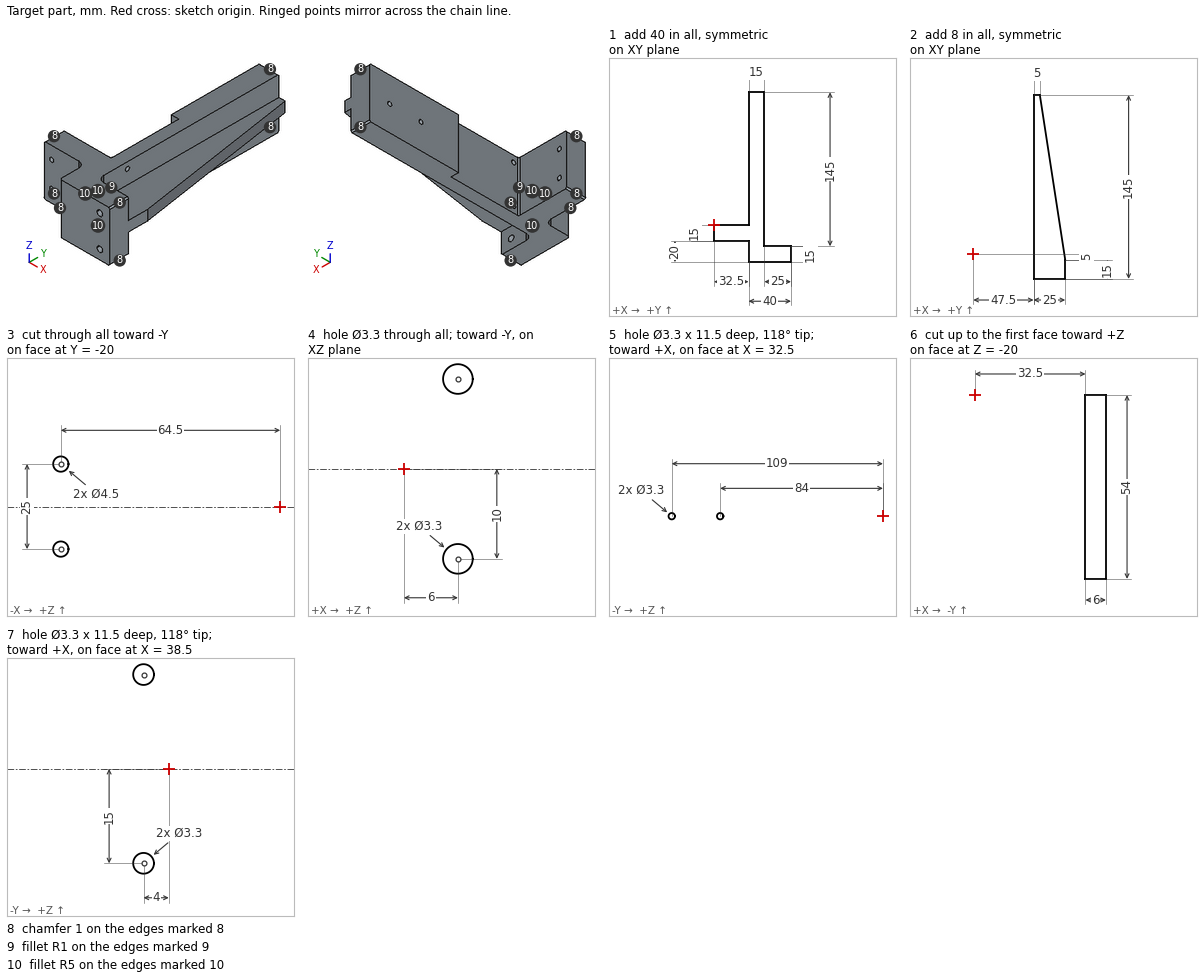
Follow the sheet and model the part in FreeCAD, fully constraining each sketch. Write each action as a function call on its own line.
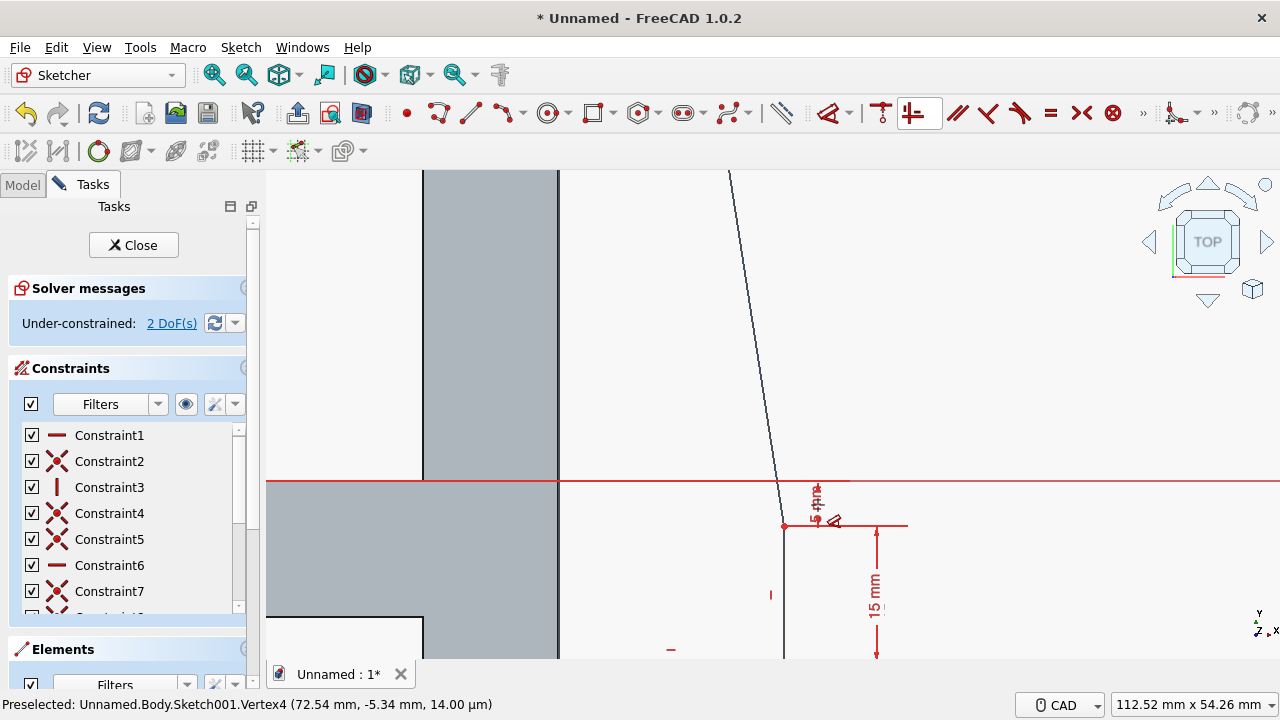
scroll(786, 547, down, 7)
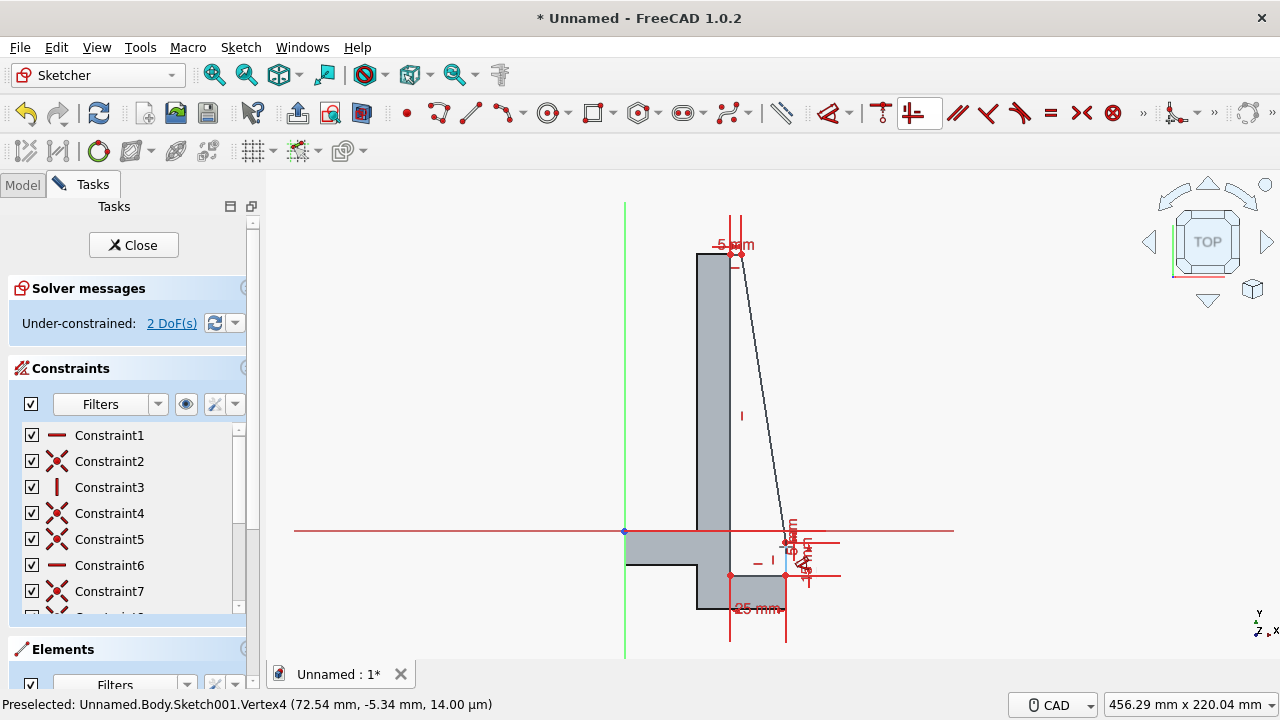
click(730, 480)
click(764, 489)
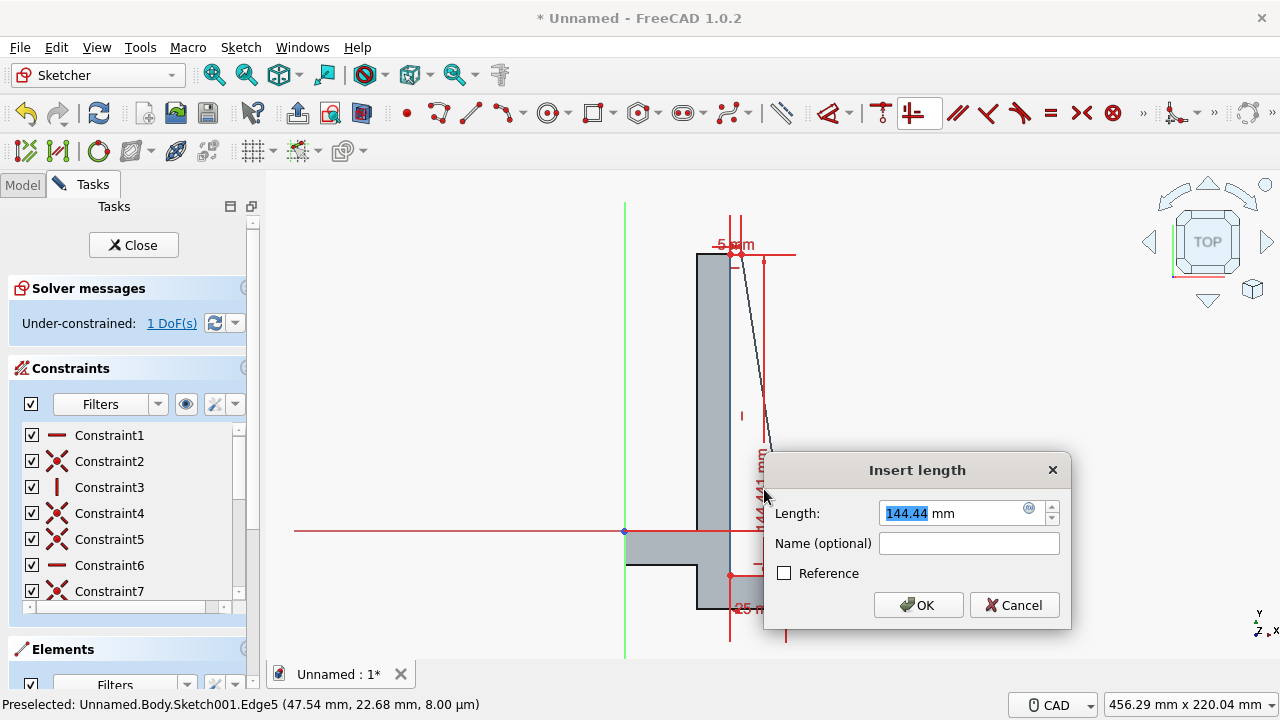
text(145)
key(Return)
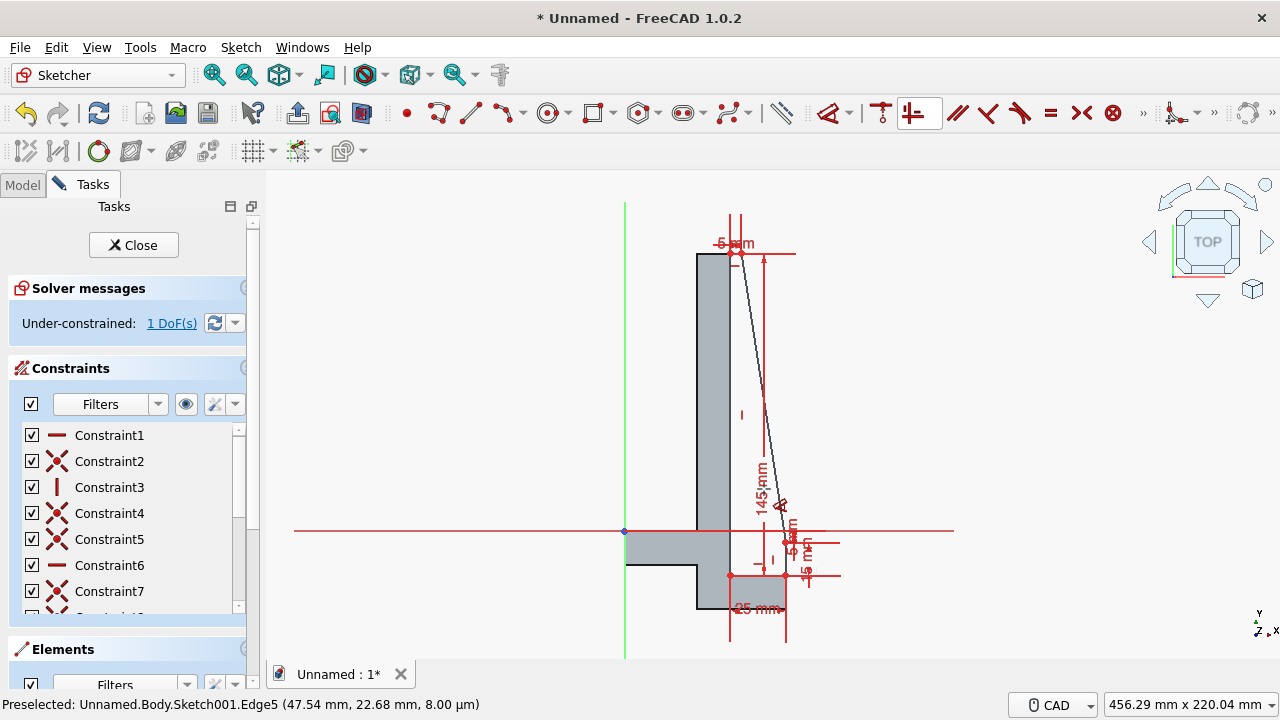
click(730, 576)
click(678, 610)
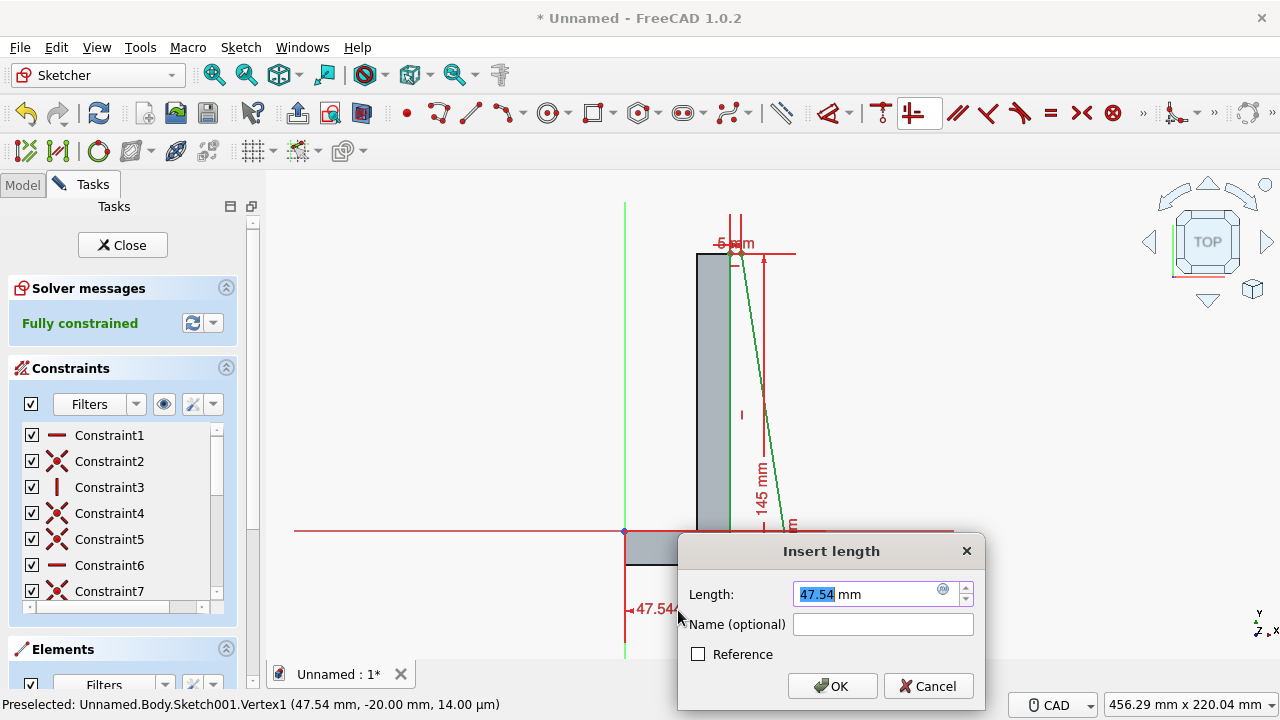
text(47.5)
key(Return)
key(Escape)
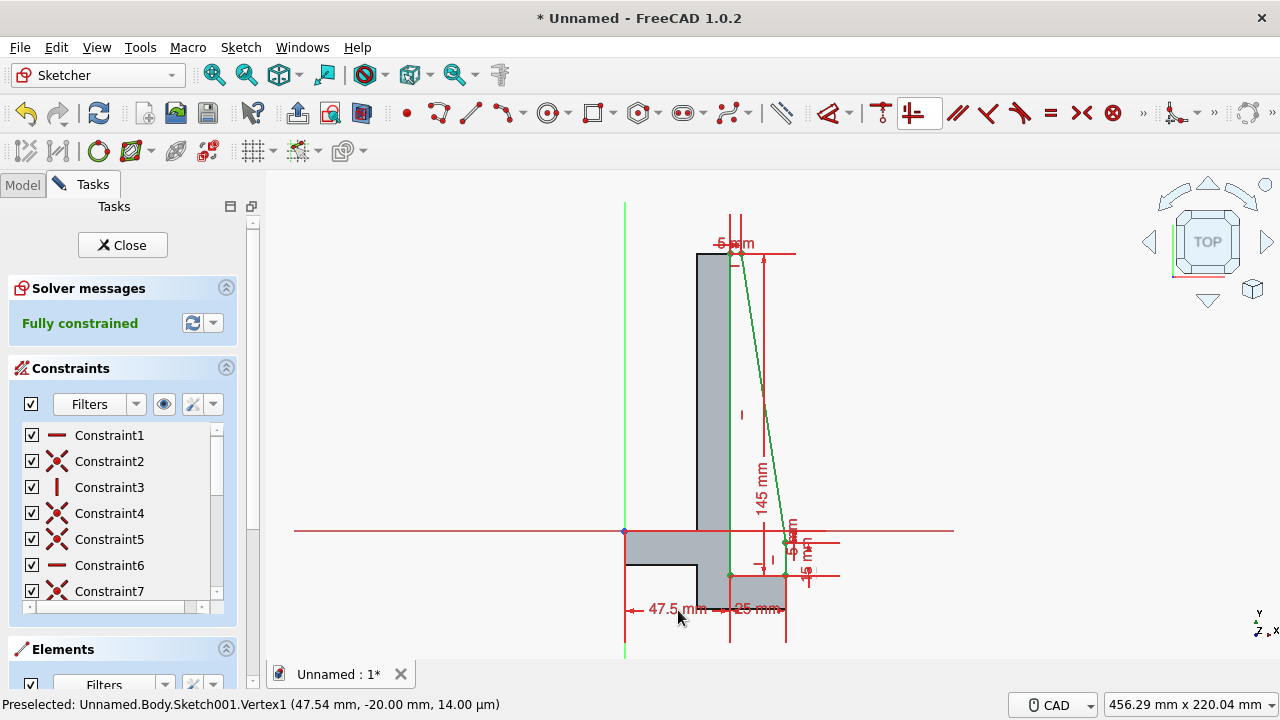
click(123, 245)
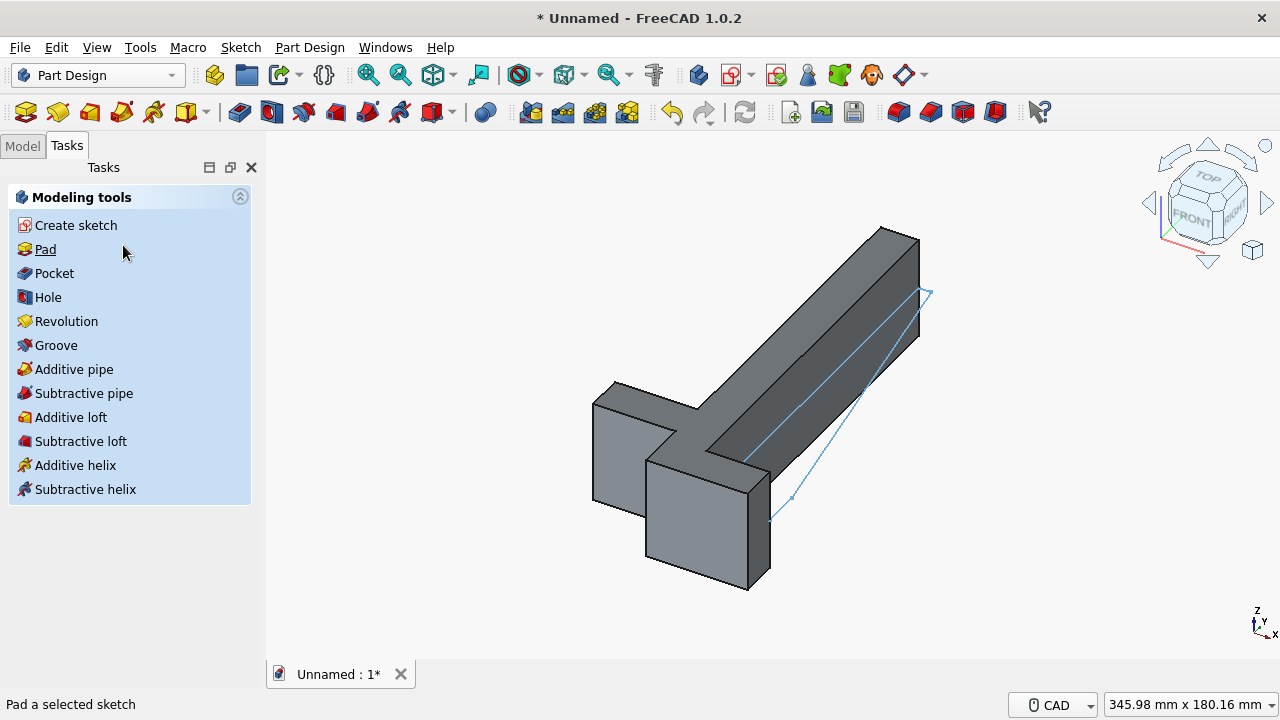
click(26, 112)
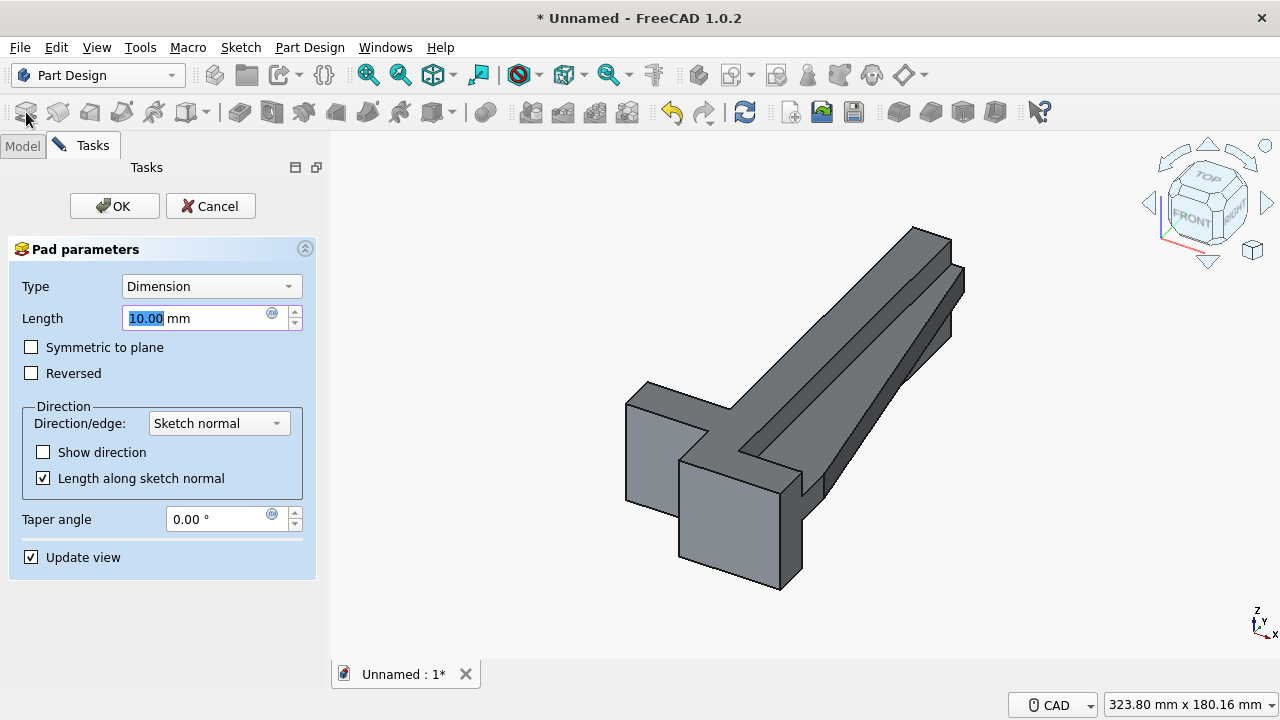
text(8)
key(Tab)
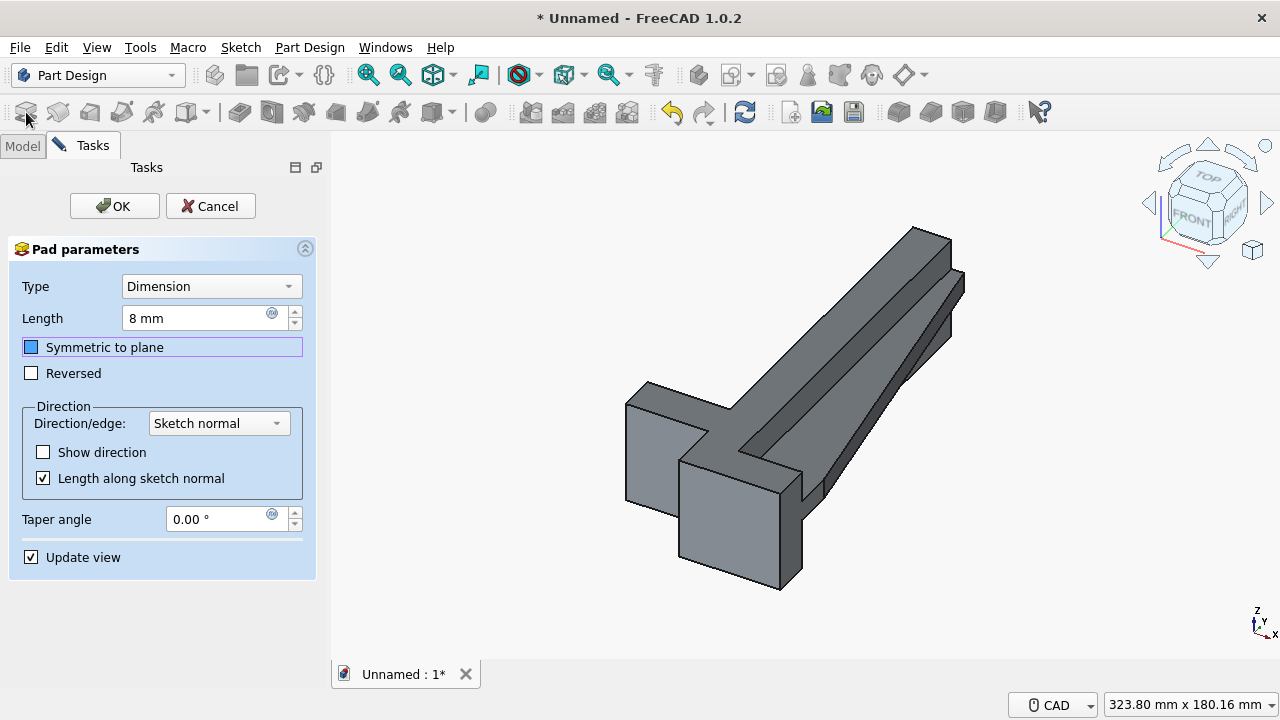
click(30, 347)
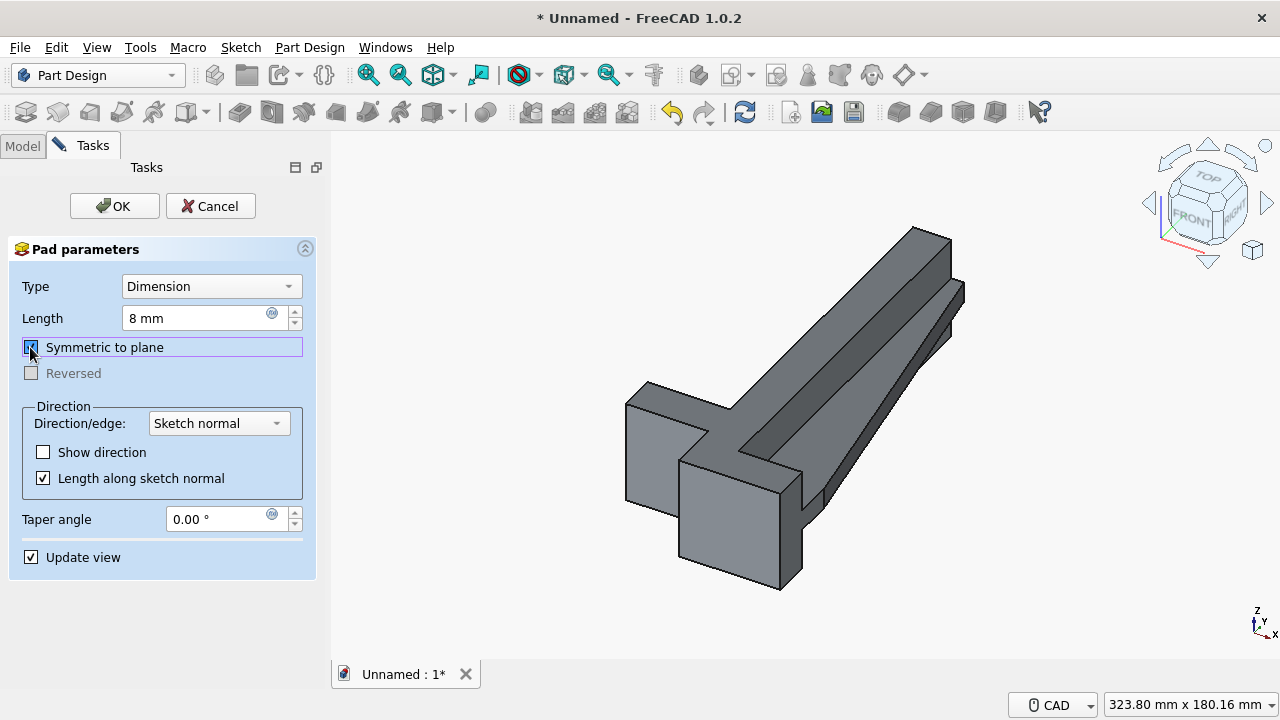
click(115, 206)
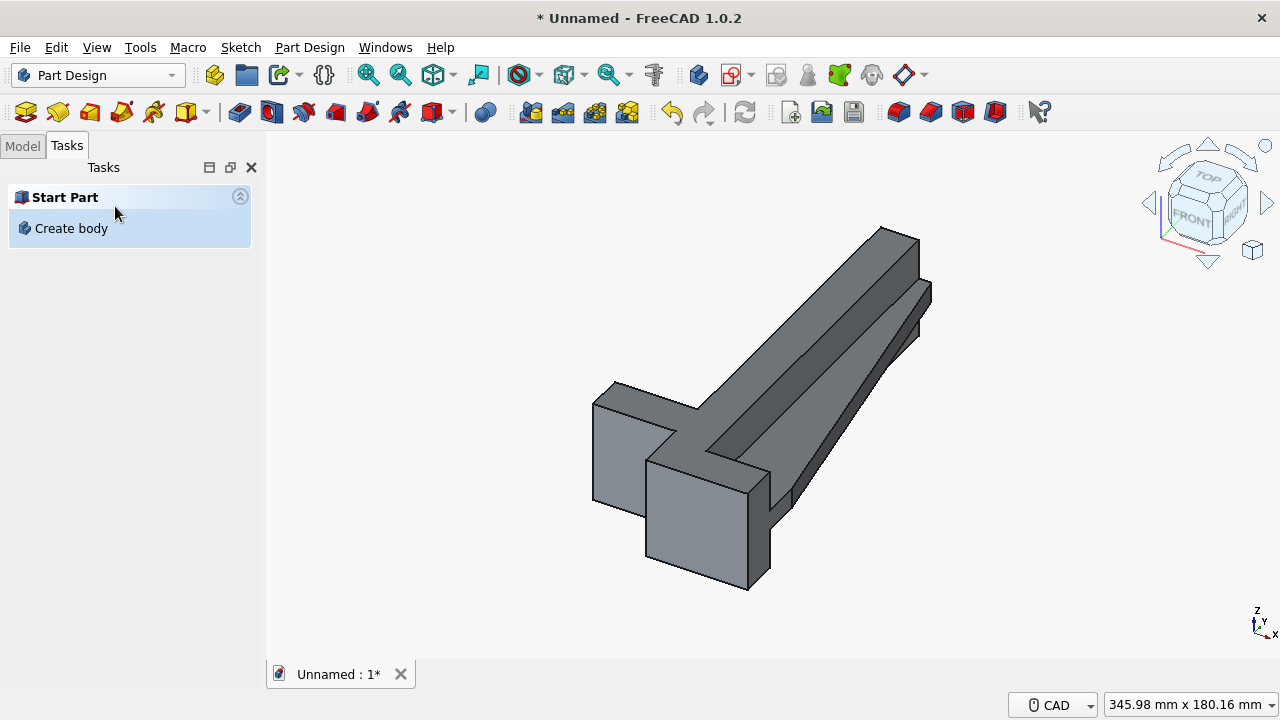
key(4)